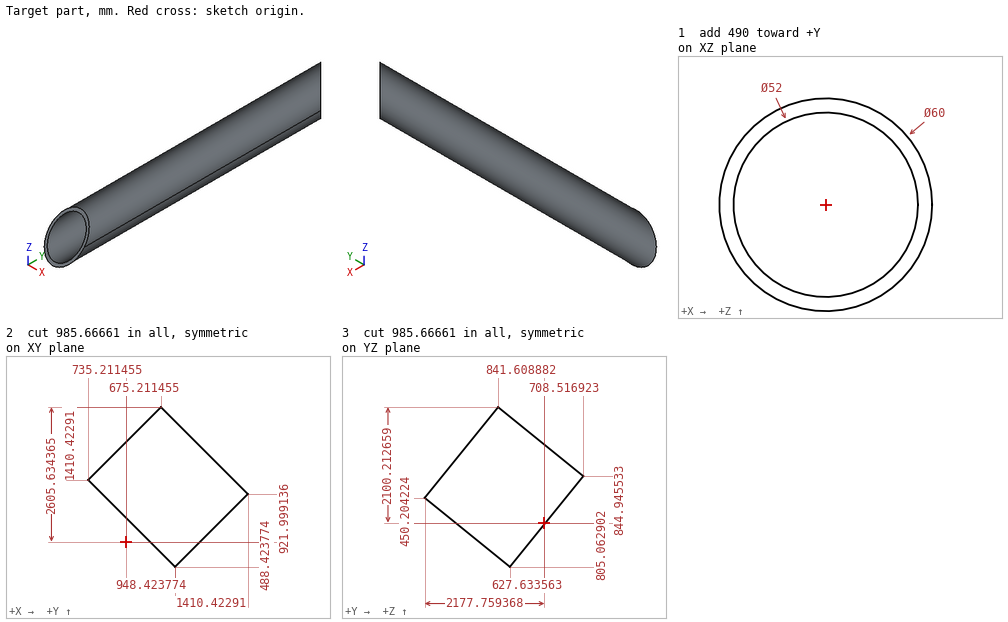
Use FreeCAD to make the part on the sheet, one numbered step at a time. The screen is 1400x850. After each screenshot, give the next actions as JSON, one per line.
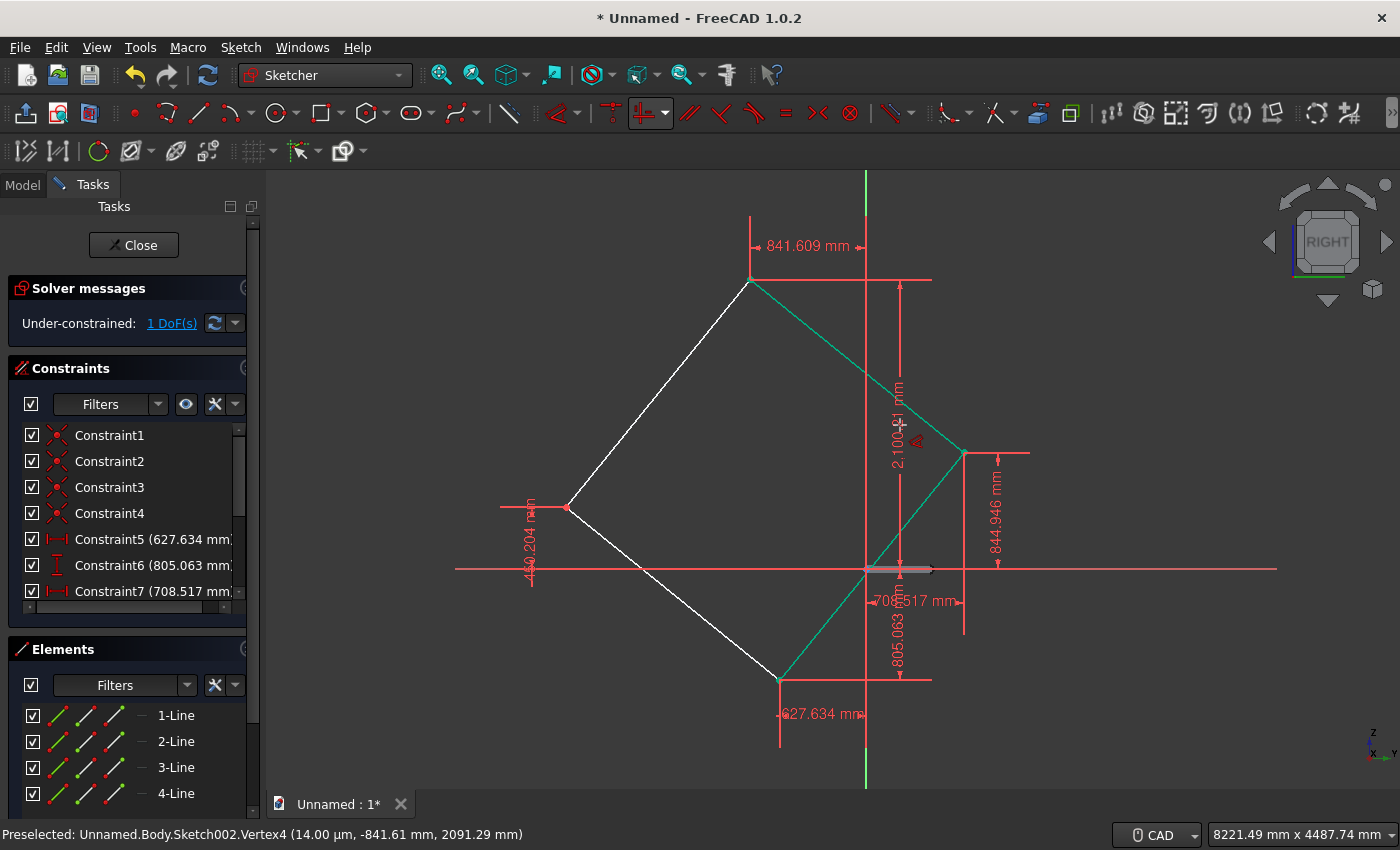
{"action": "left_click", "coordinate": [566, 507]}
{"action": "left_click", "coordinate": [716, 603]}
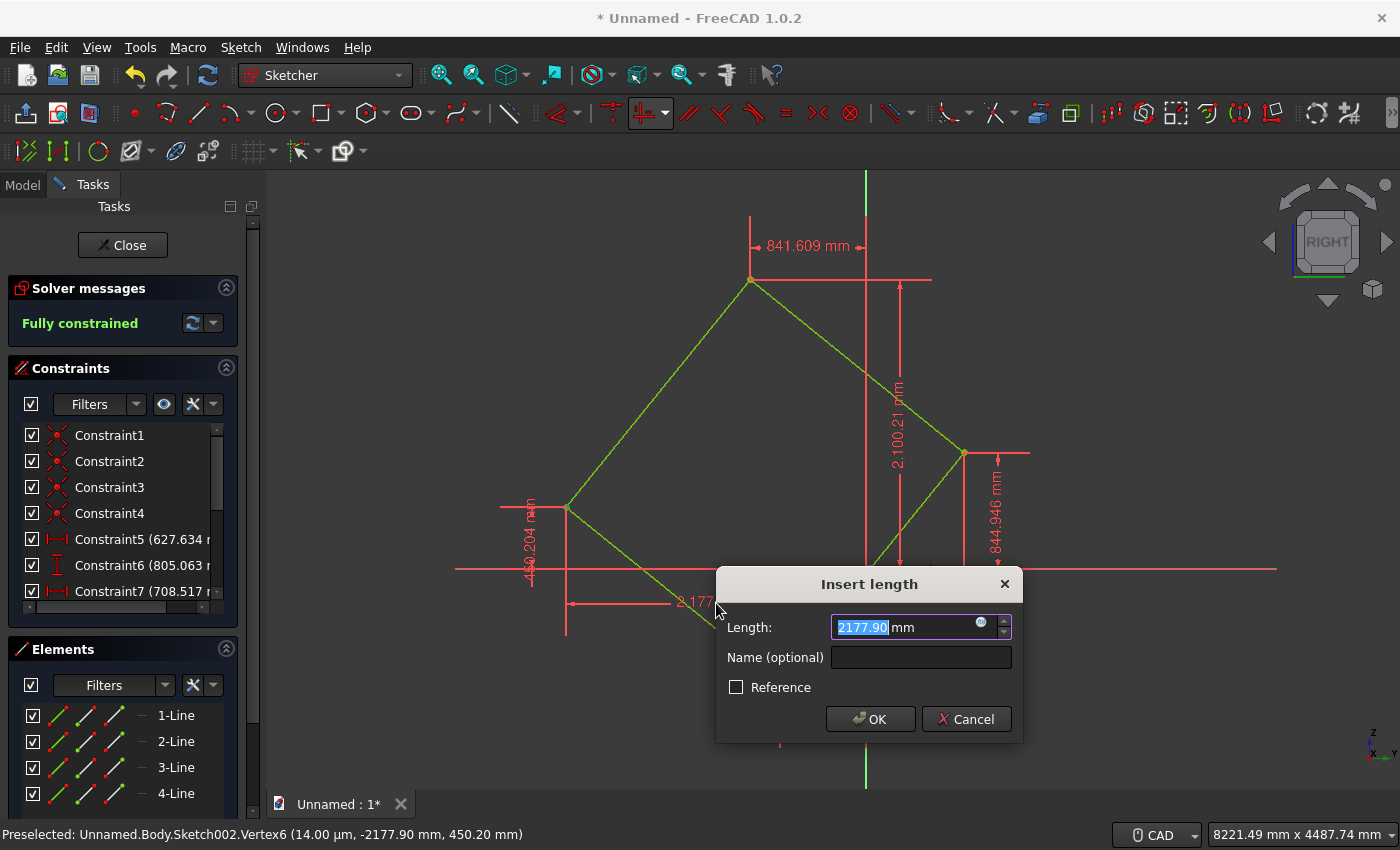
{"action": "type", "text": "2177.759368"}
{"action": "key", "text": "Return"}
{"action": "key", "text": "Escape"}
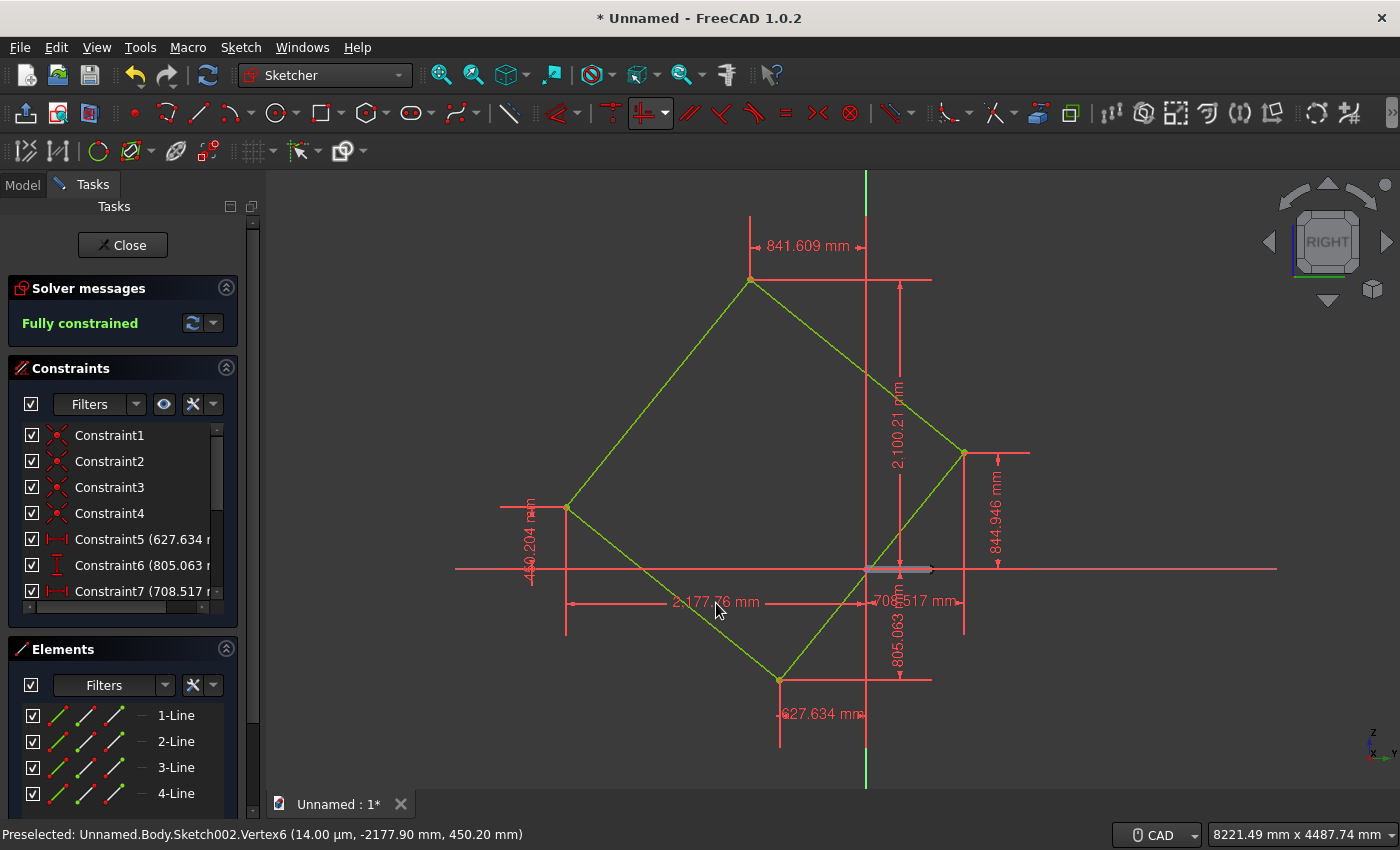
{"action": "left_click", "coordinate": [123, 245]}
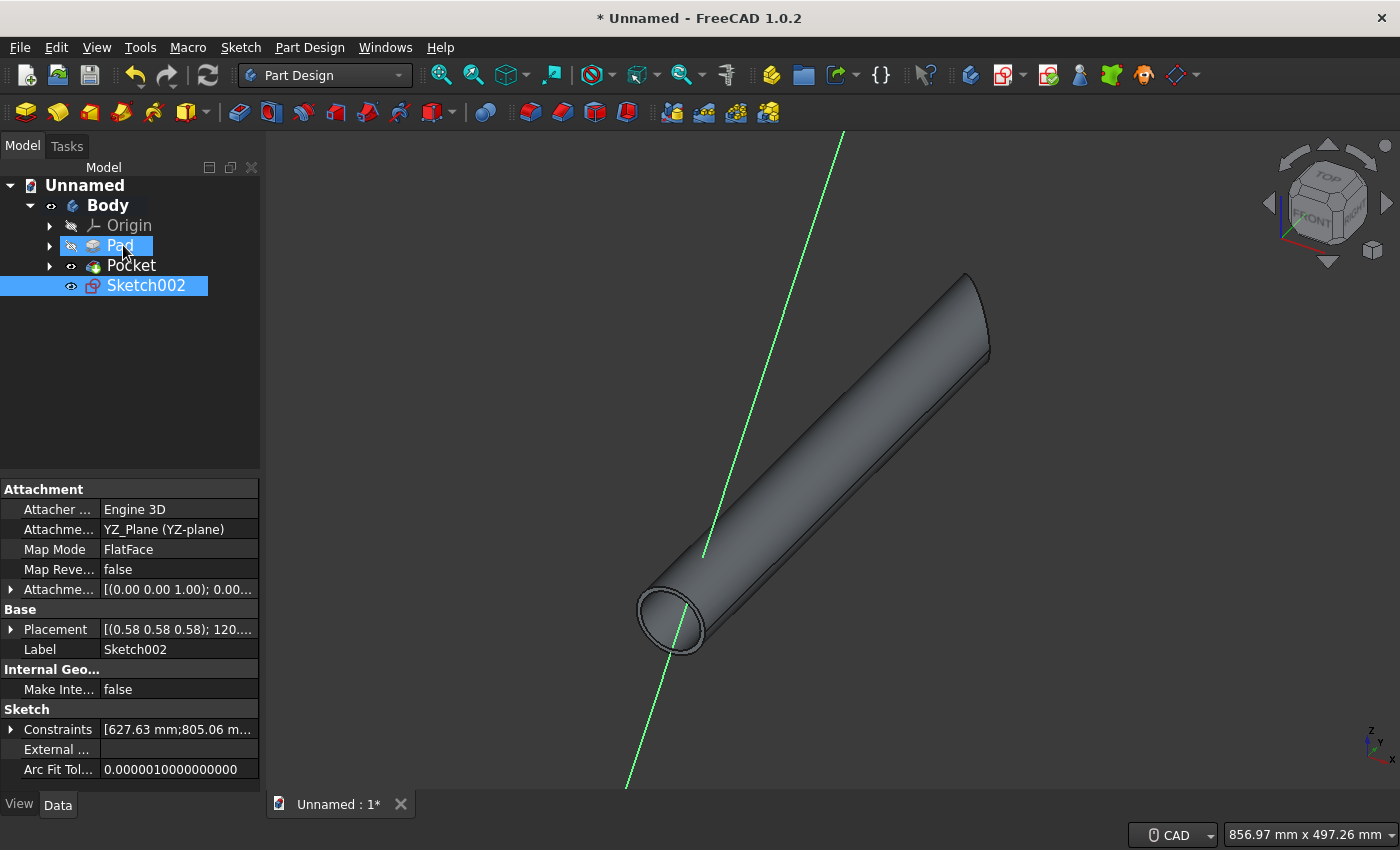
{"action": "left_click", "coordinate": [240, 112]}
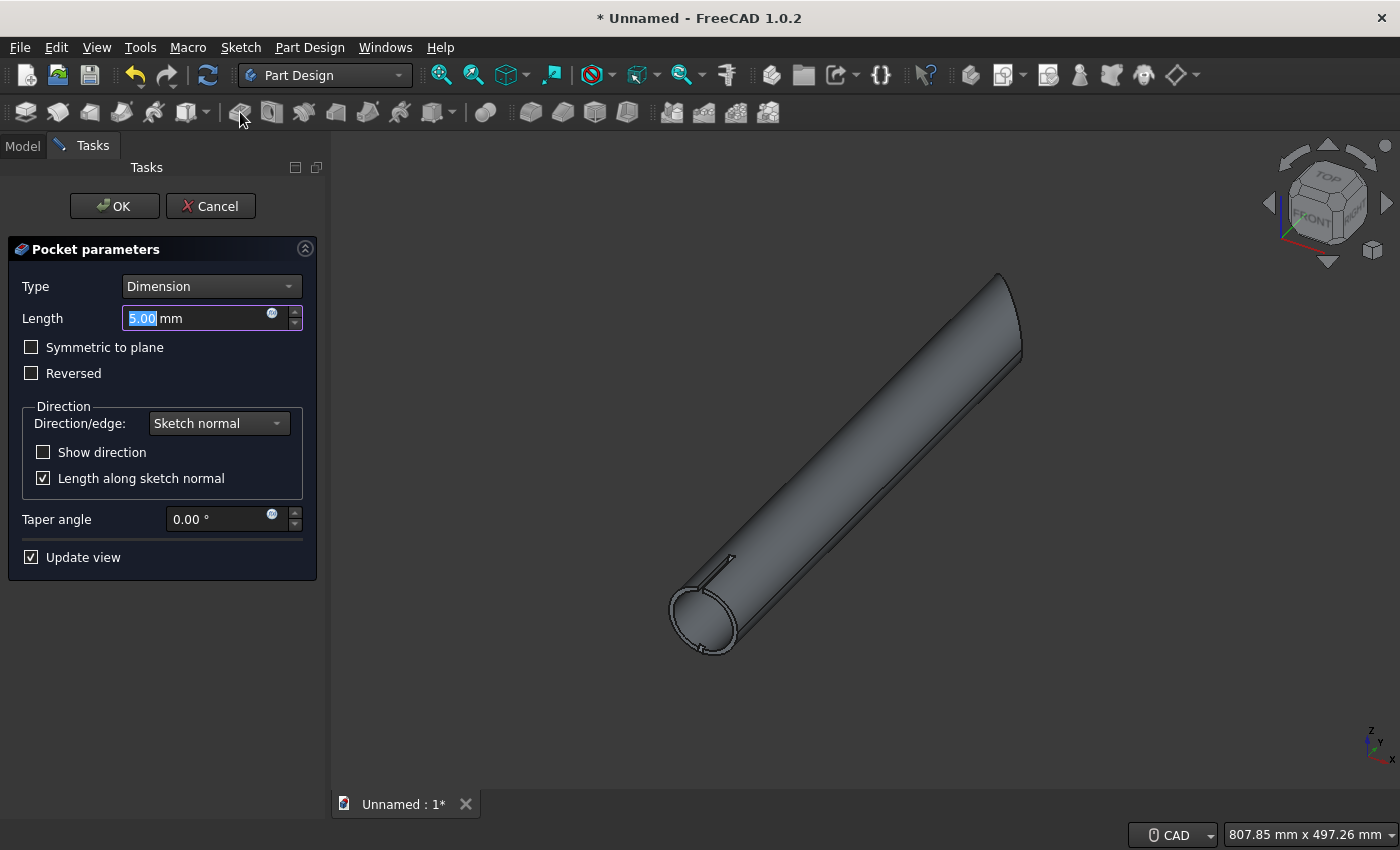
{"action": "type", "text": "985.66661"}
{"action": "key", "text": "Tab"}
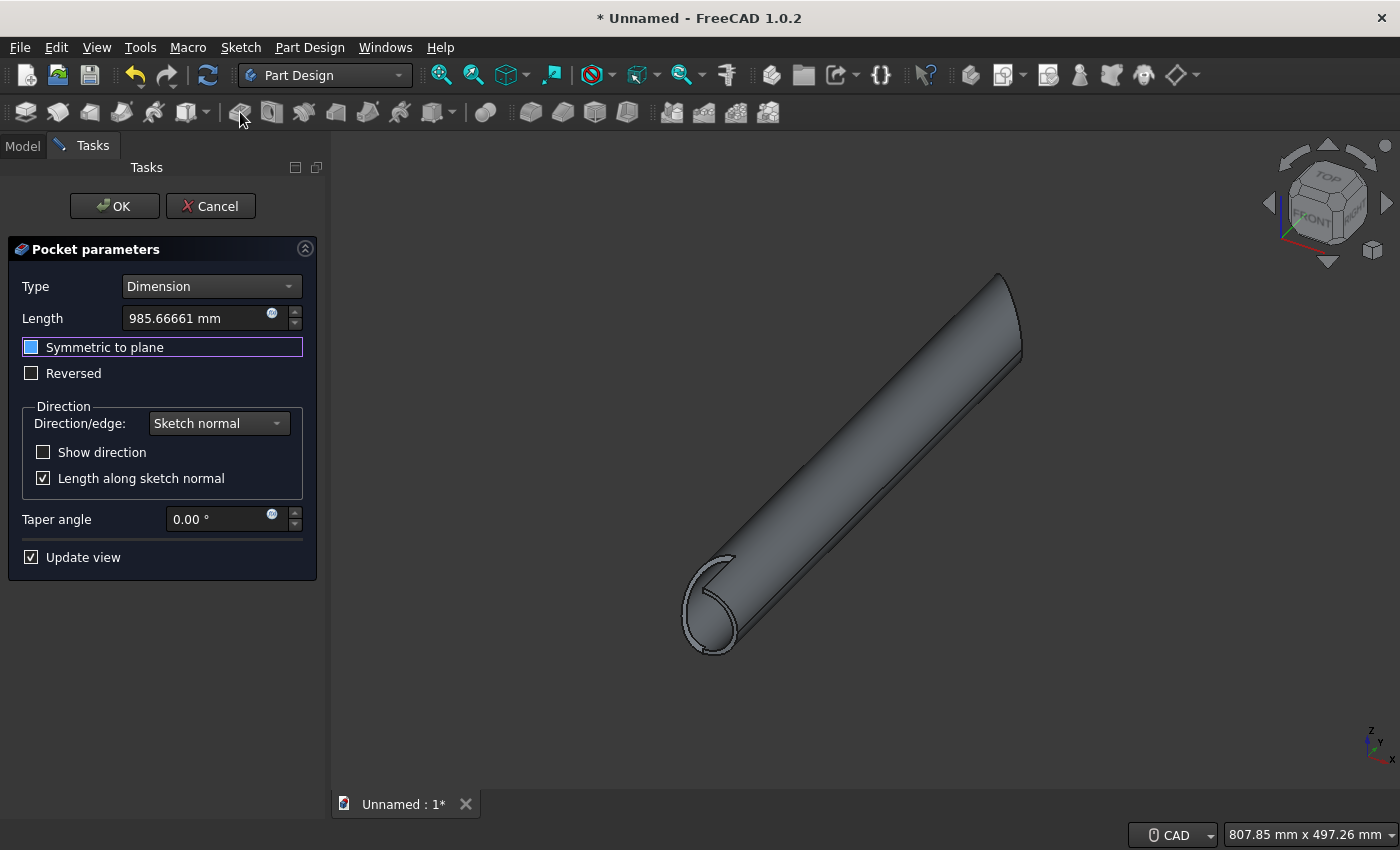
{"action": "left_click", "coordinate": [30, 347]}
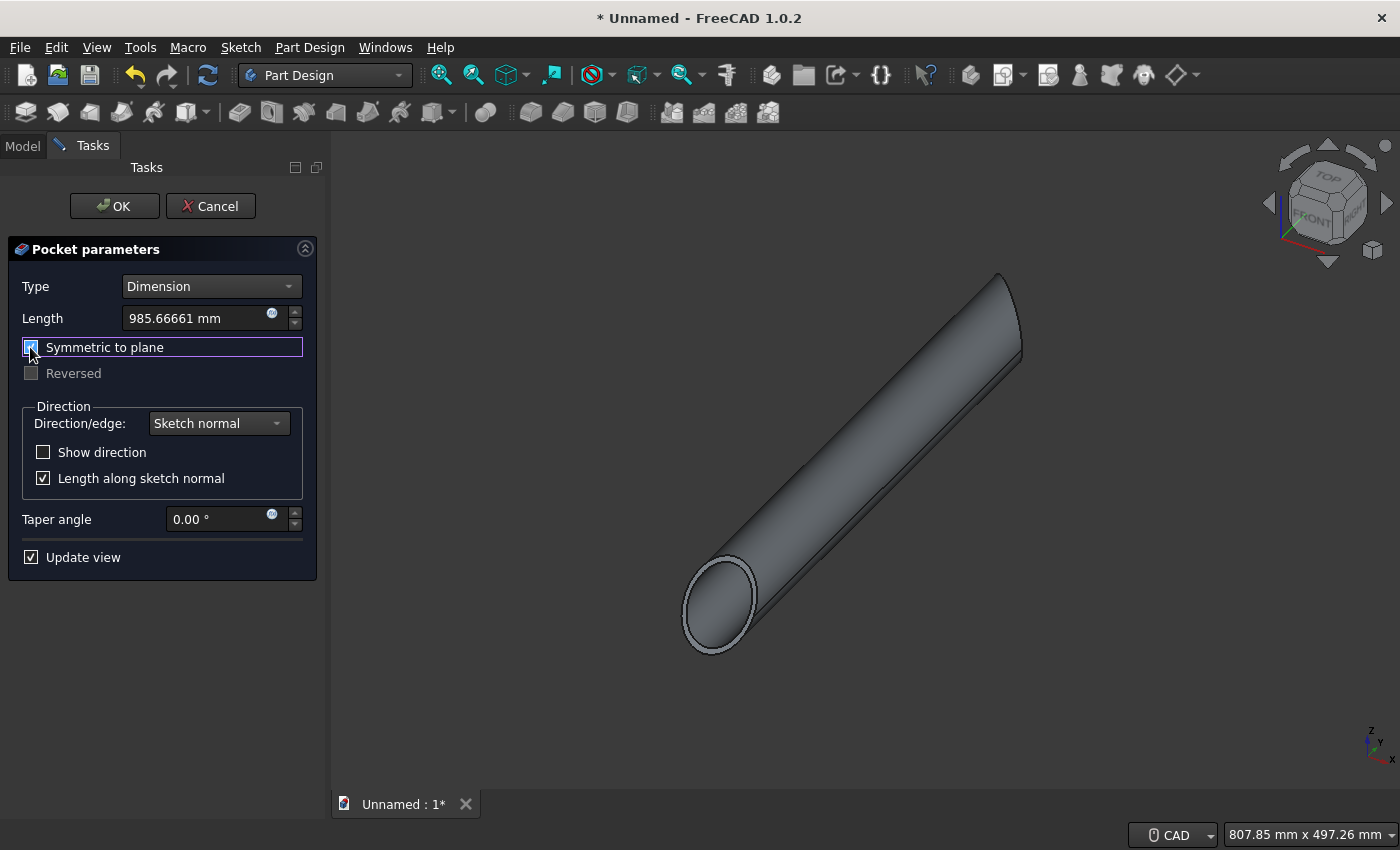
{"action": "left_click", "coordinate": [115, 206]}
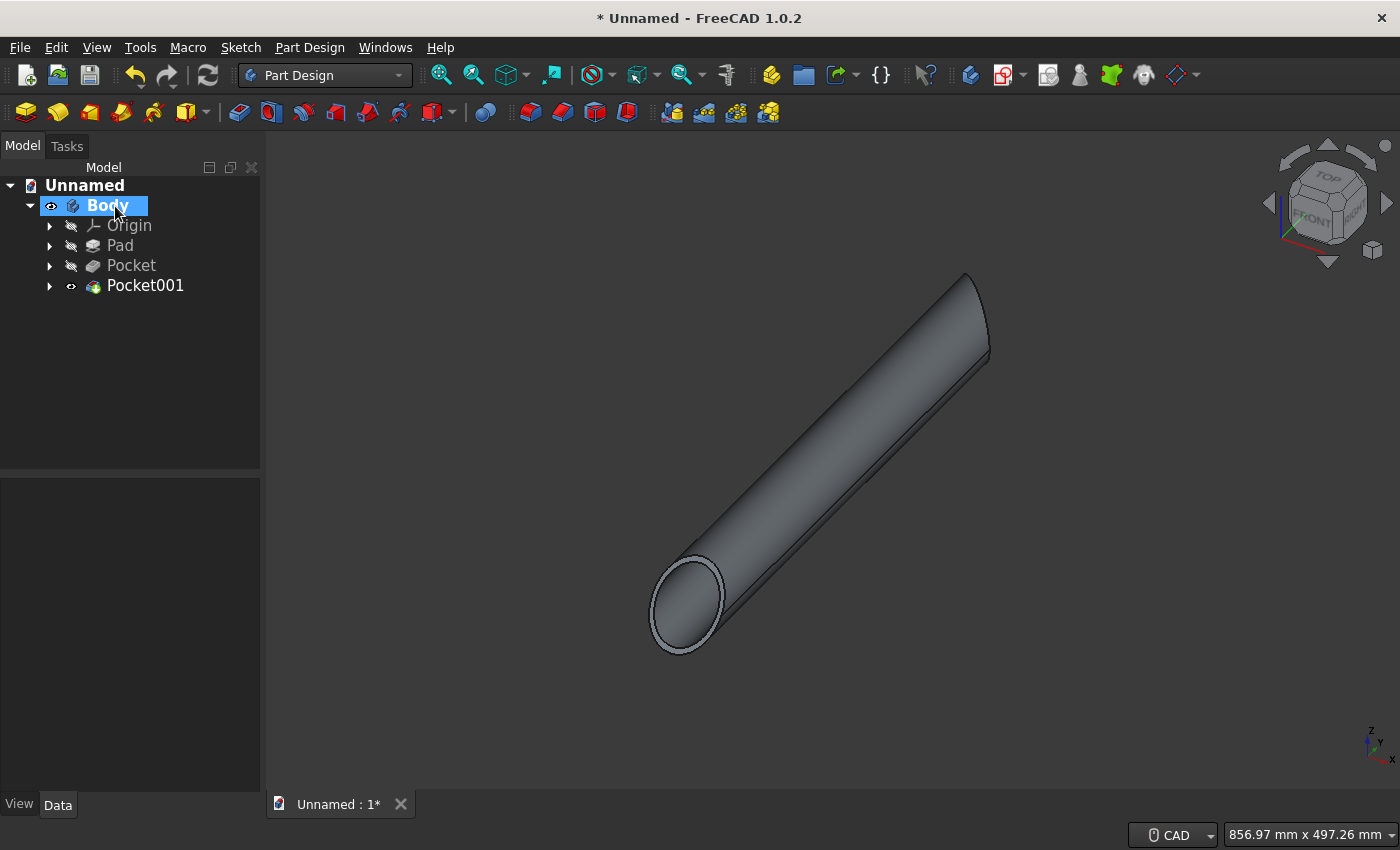
{"action": "key", "text": "0"}